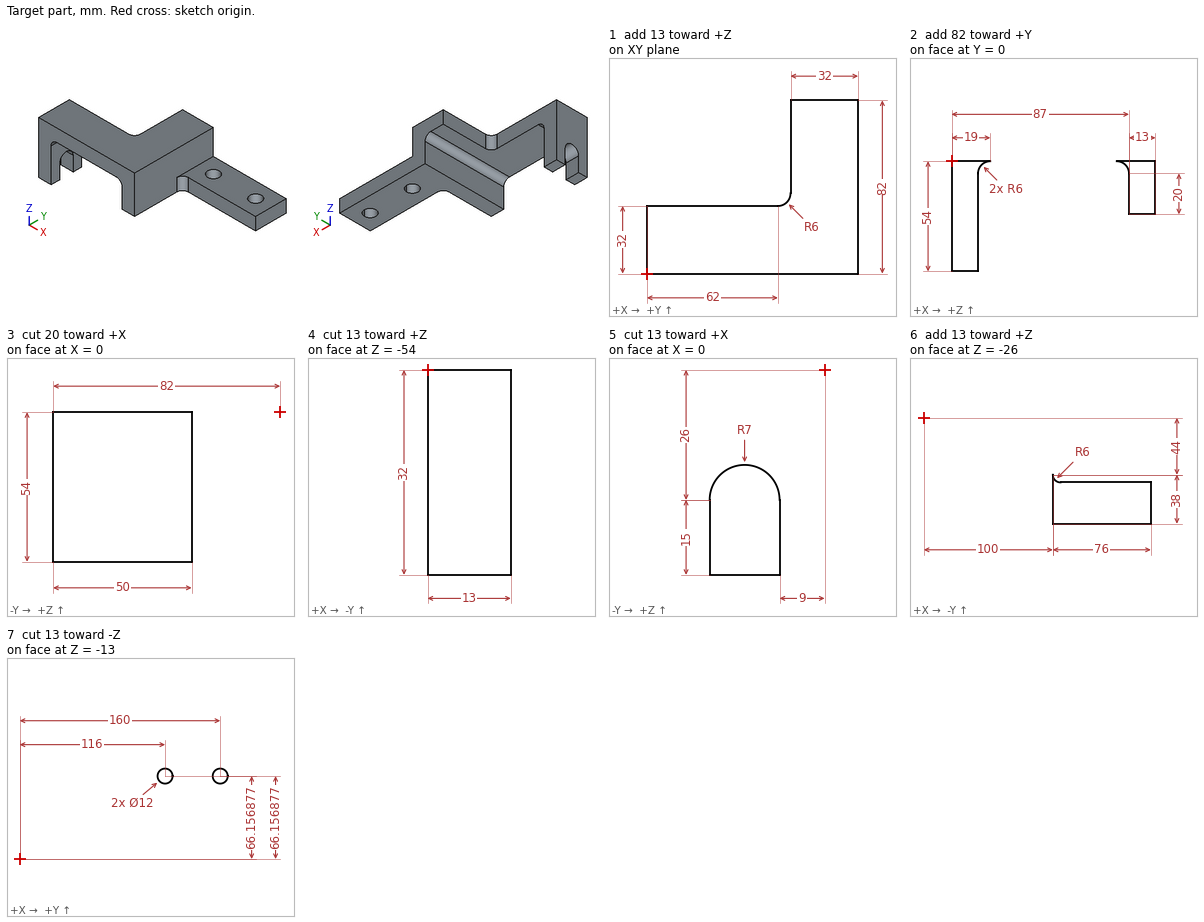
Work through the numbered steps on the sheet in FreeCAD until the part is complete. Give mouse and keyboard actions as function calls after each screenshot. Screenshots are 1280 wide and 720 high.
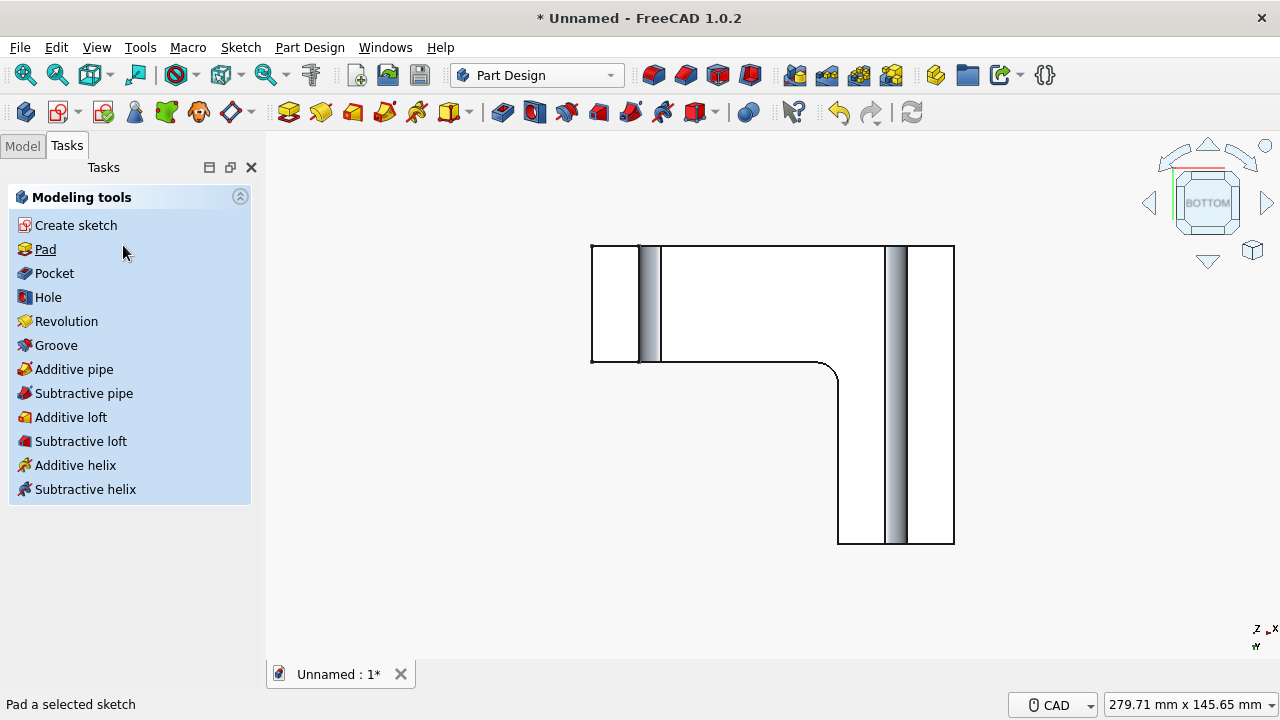
click(504, 112)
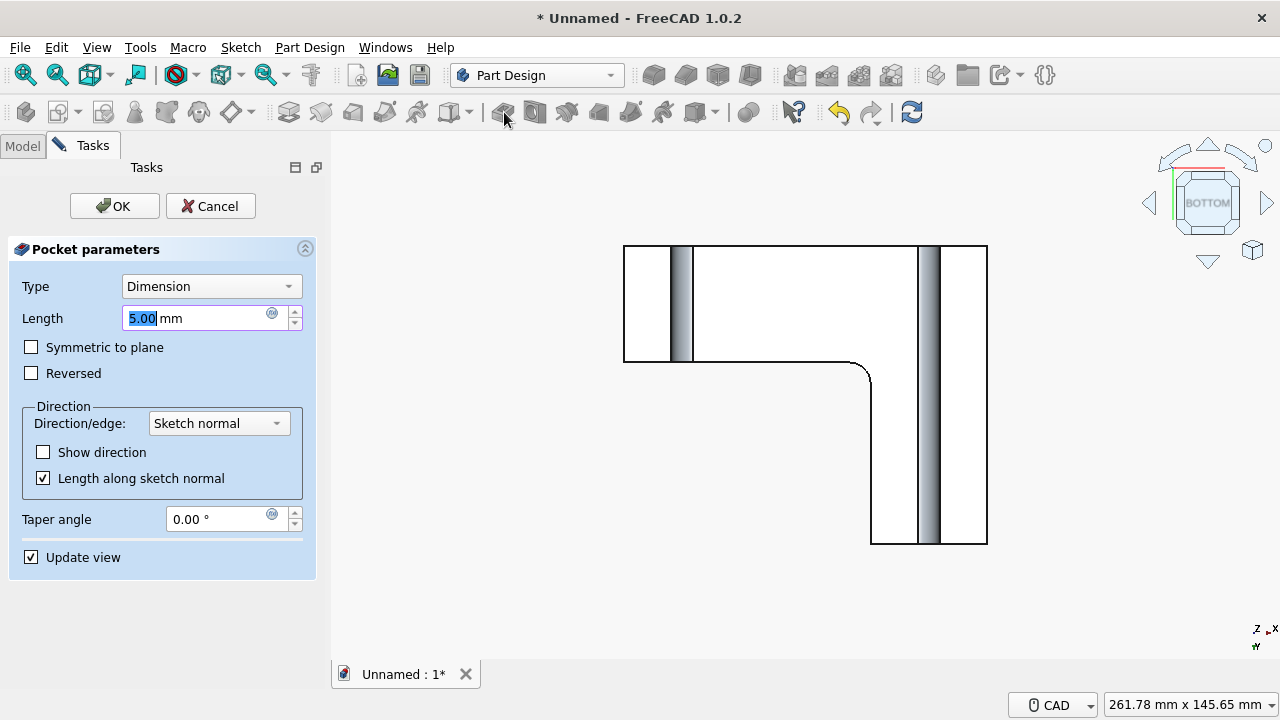
text(13)
key(Tab)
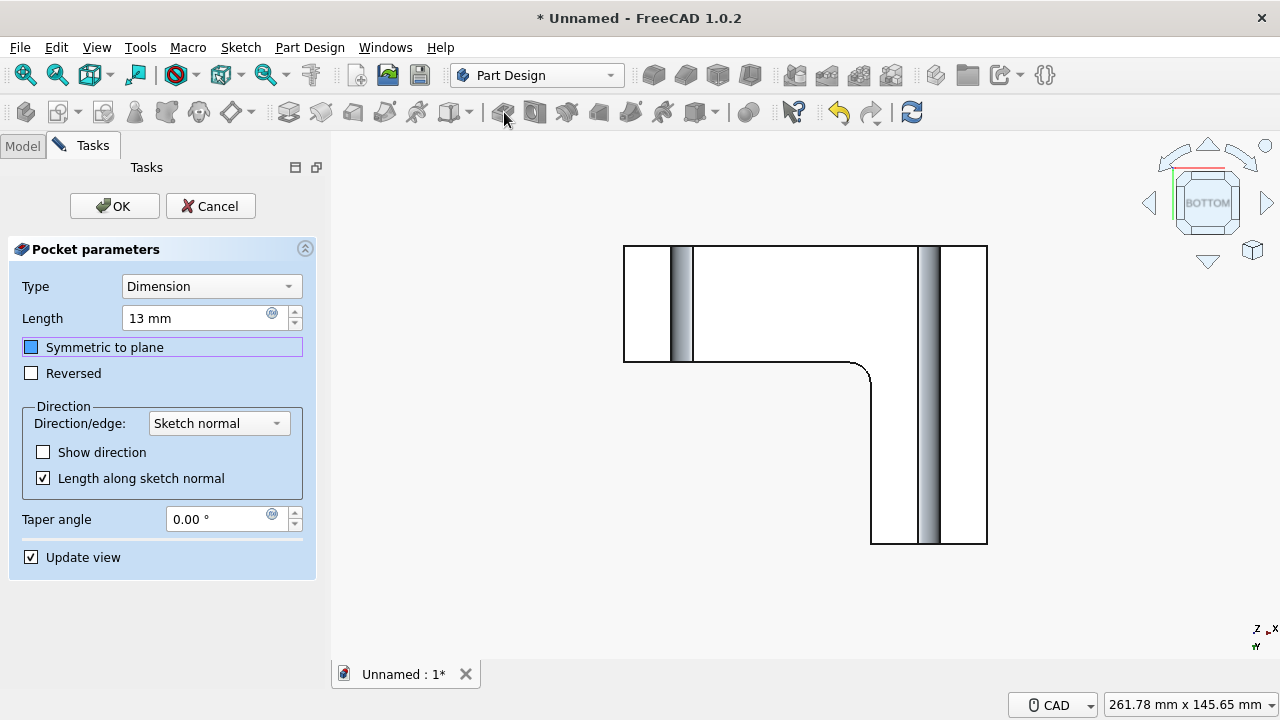
click(115, 206)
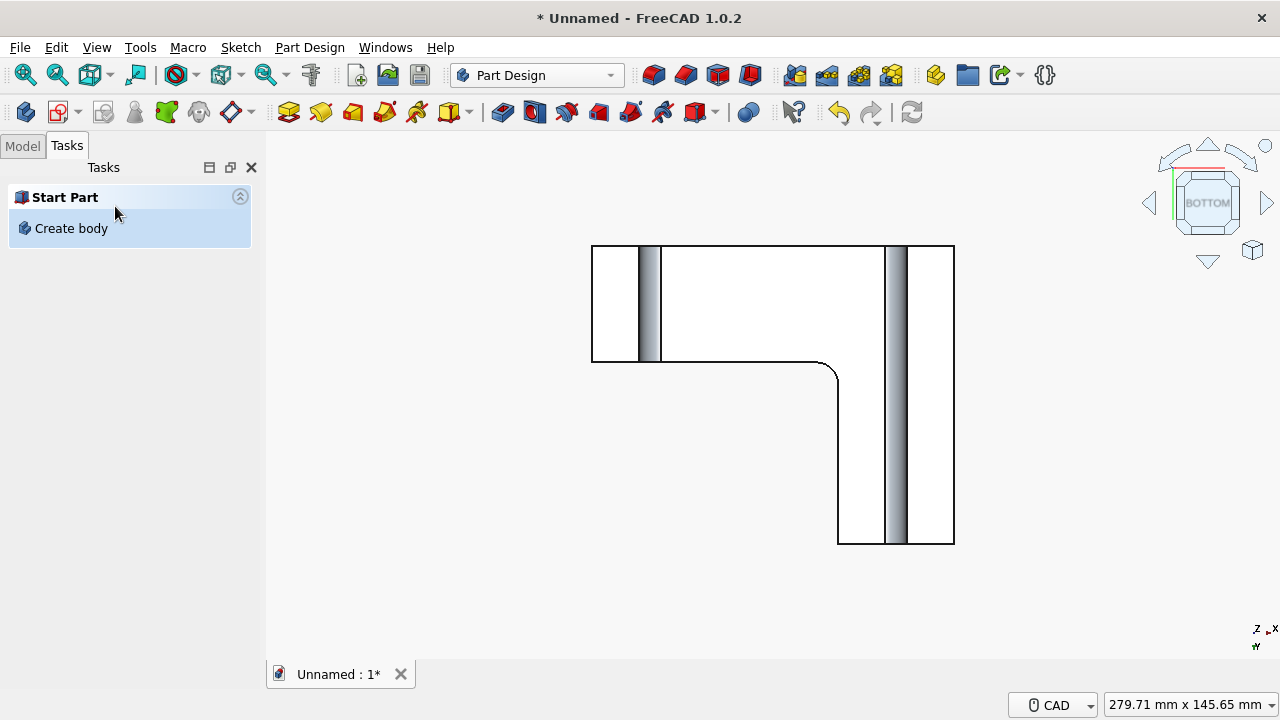
key(6)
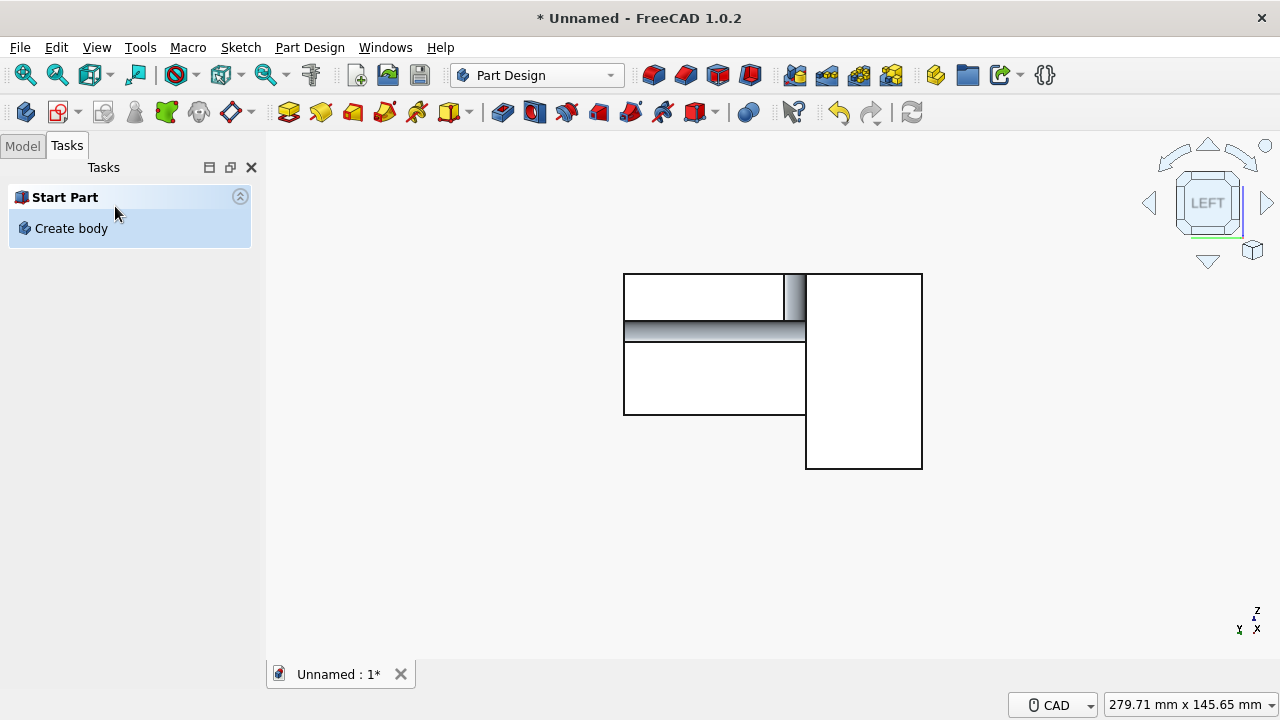
click(26, 76)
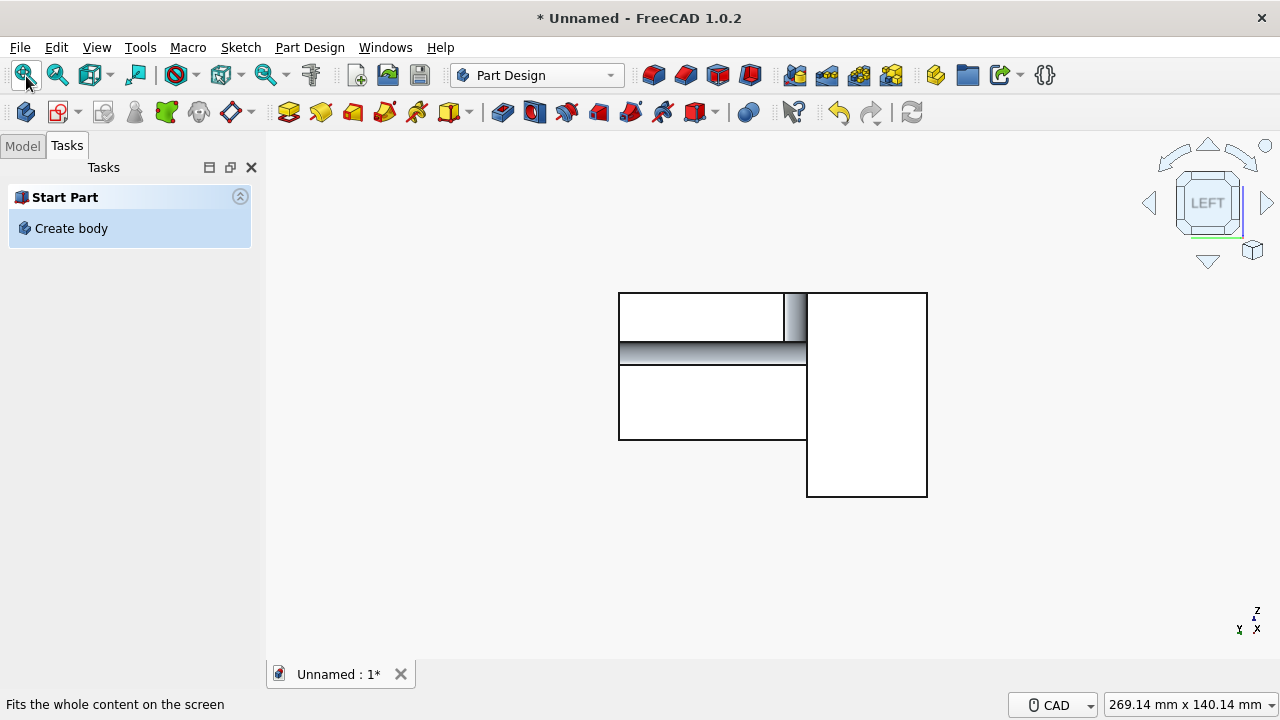
click(867, 423)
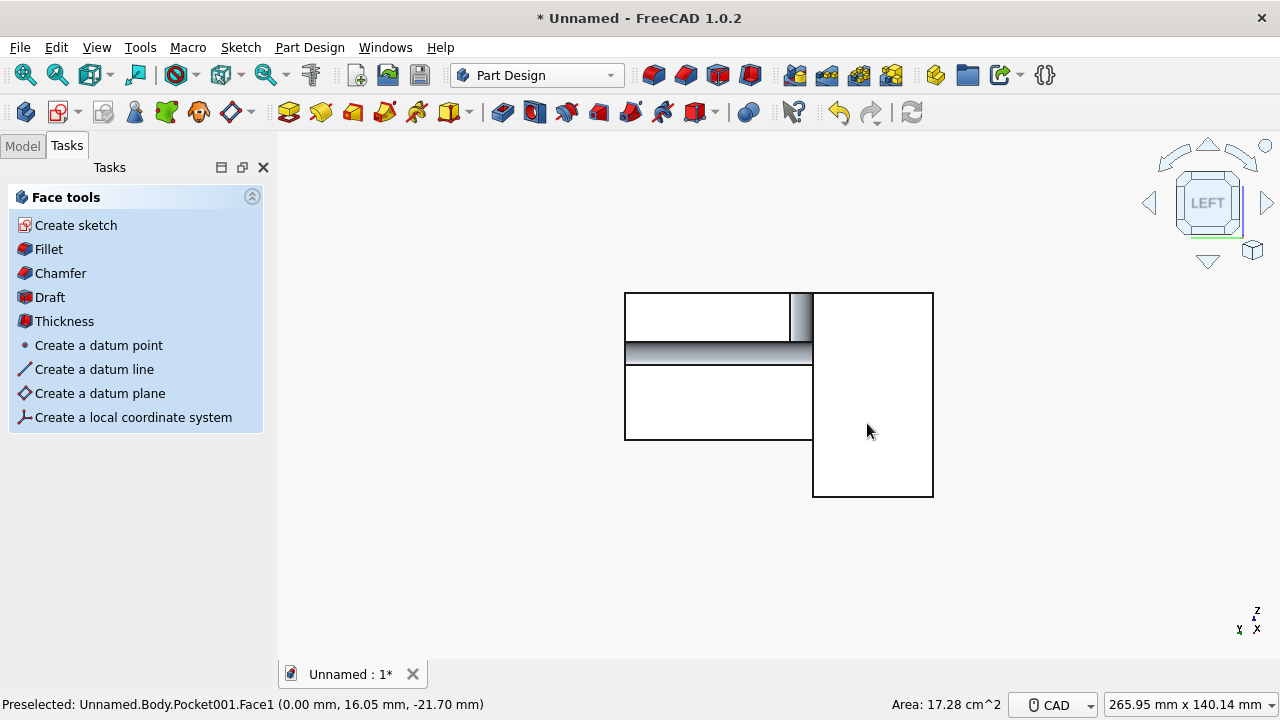
click(58, 112)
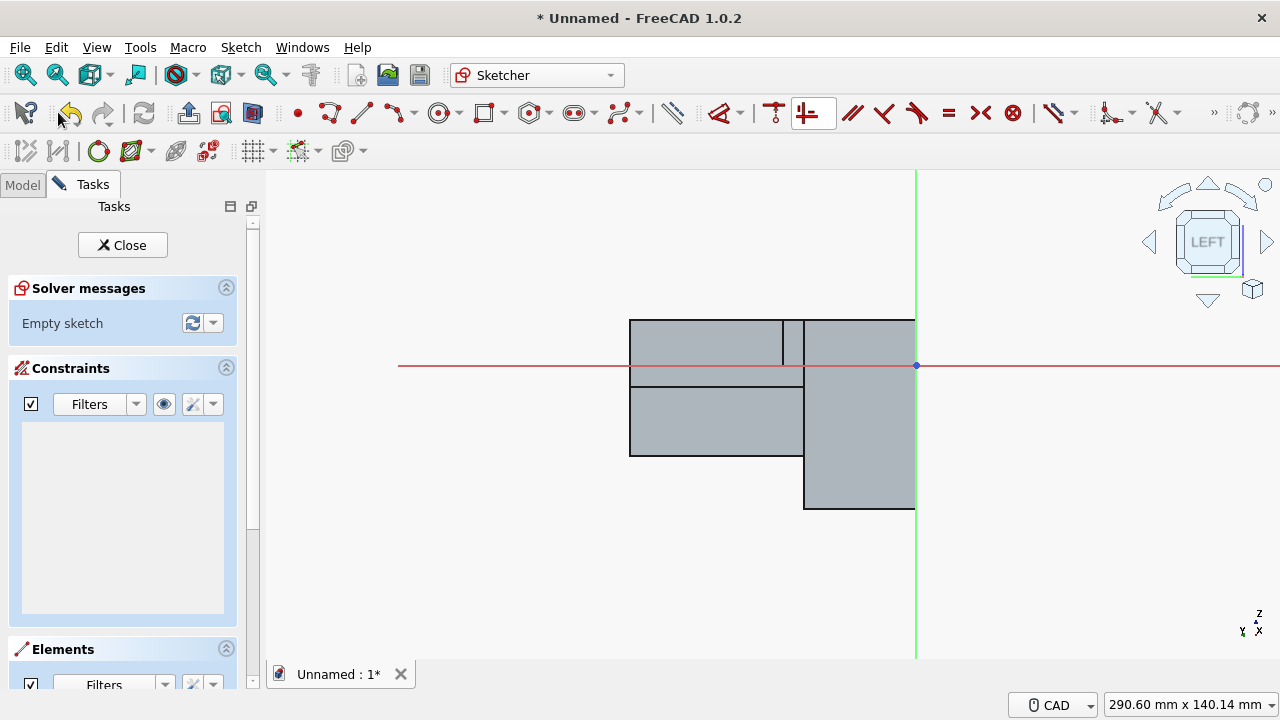
scroll(1016, 456, up, 4)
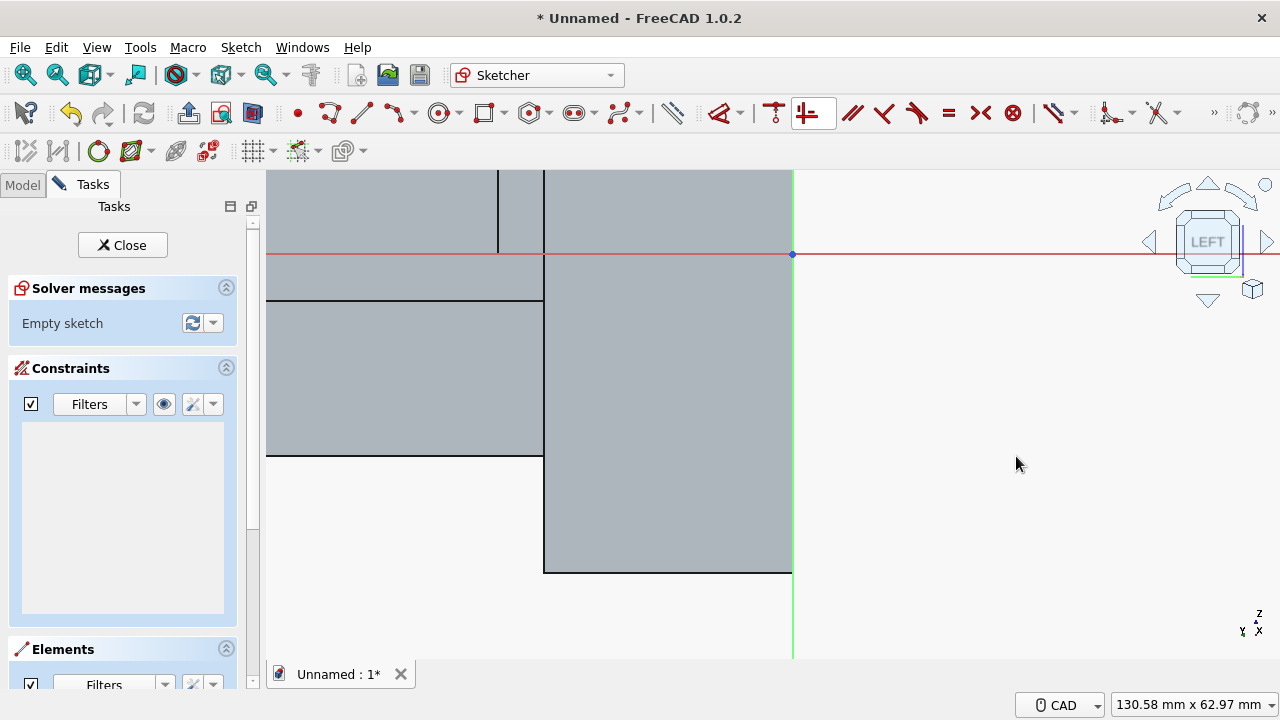
click(330, 114)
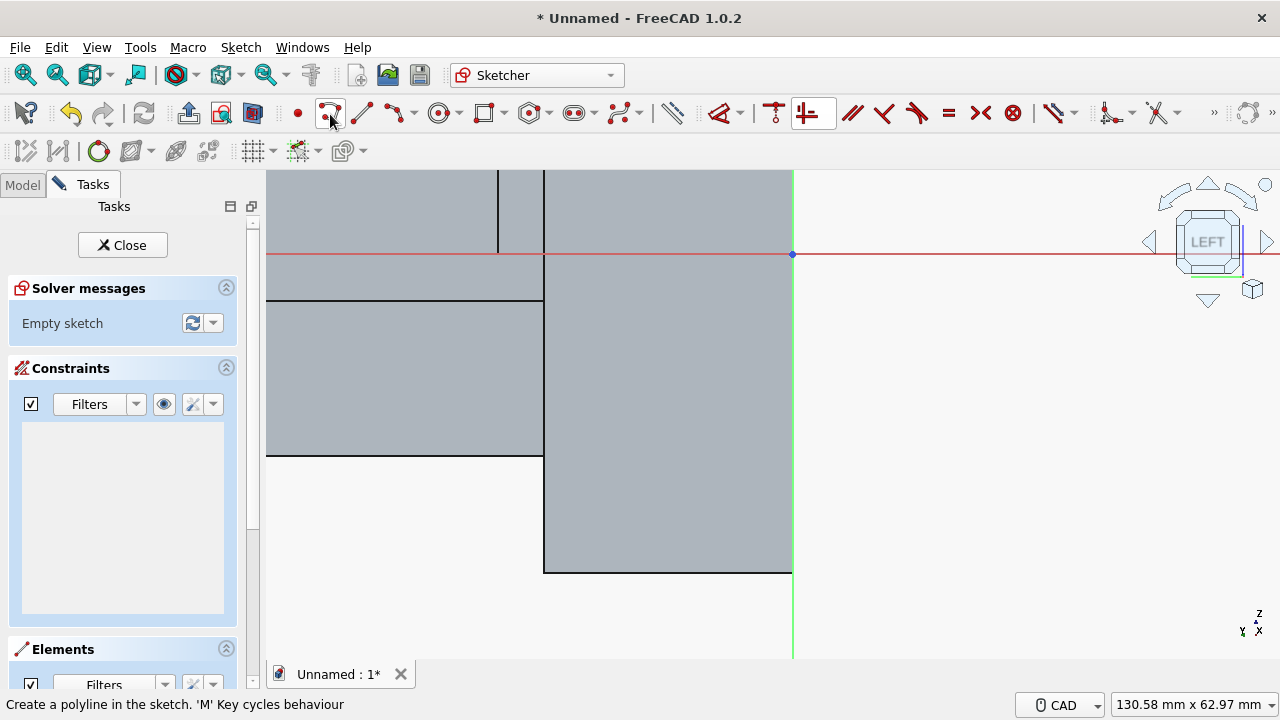
click(614, 456)
click(614, 573)
click(723, 573)
click(723, 456)
right_click(723, 456)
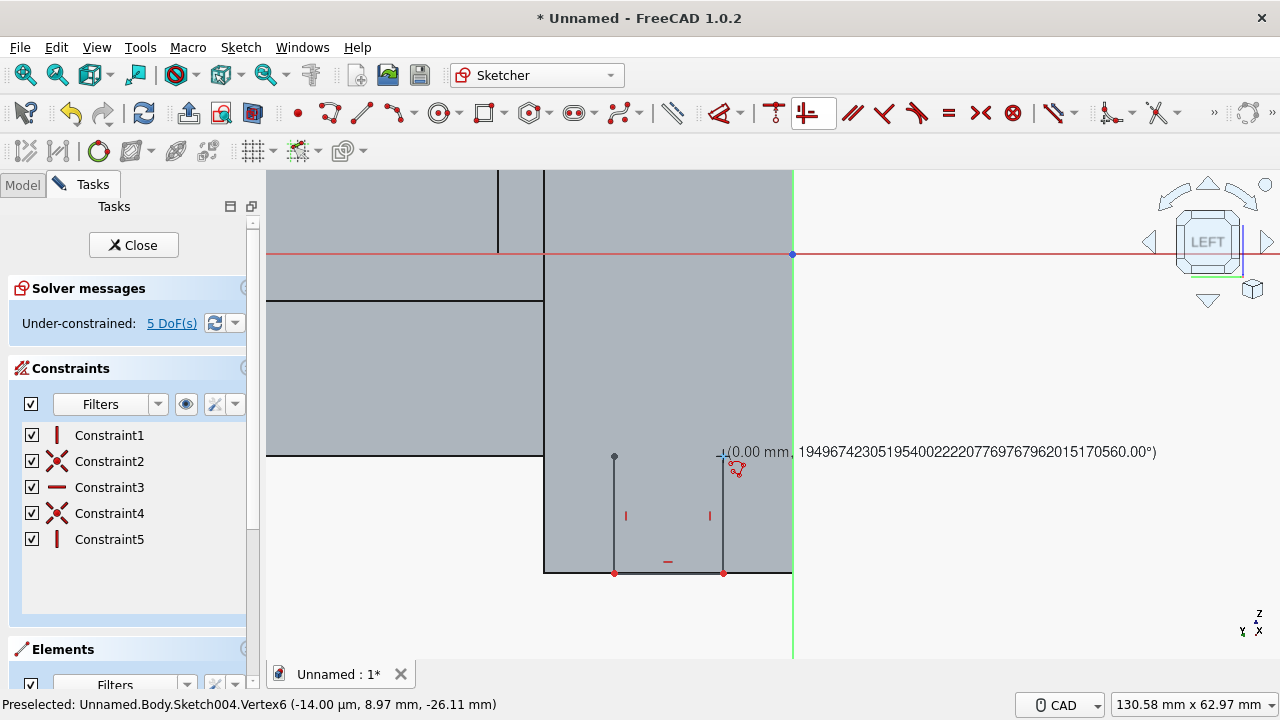
click(394, 114)